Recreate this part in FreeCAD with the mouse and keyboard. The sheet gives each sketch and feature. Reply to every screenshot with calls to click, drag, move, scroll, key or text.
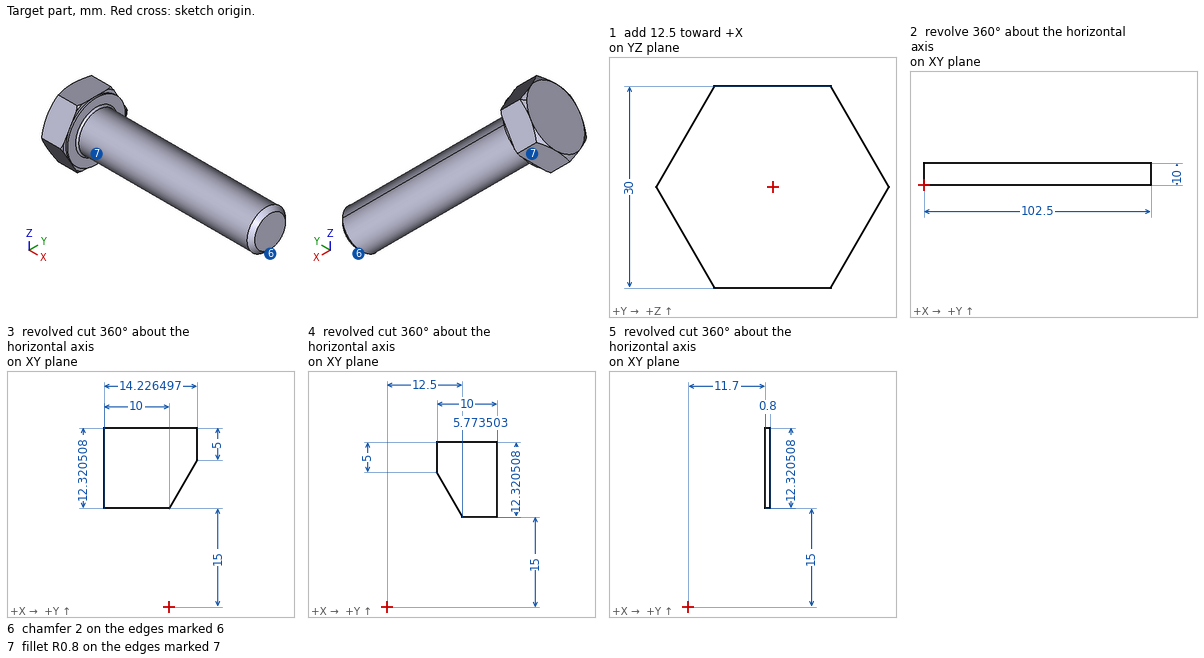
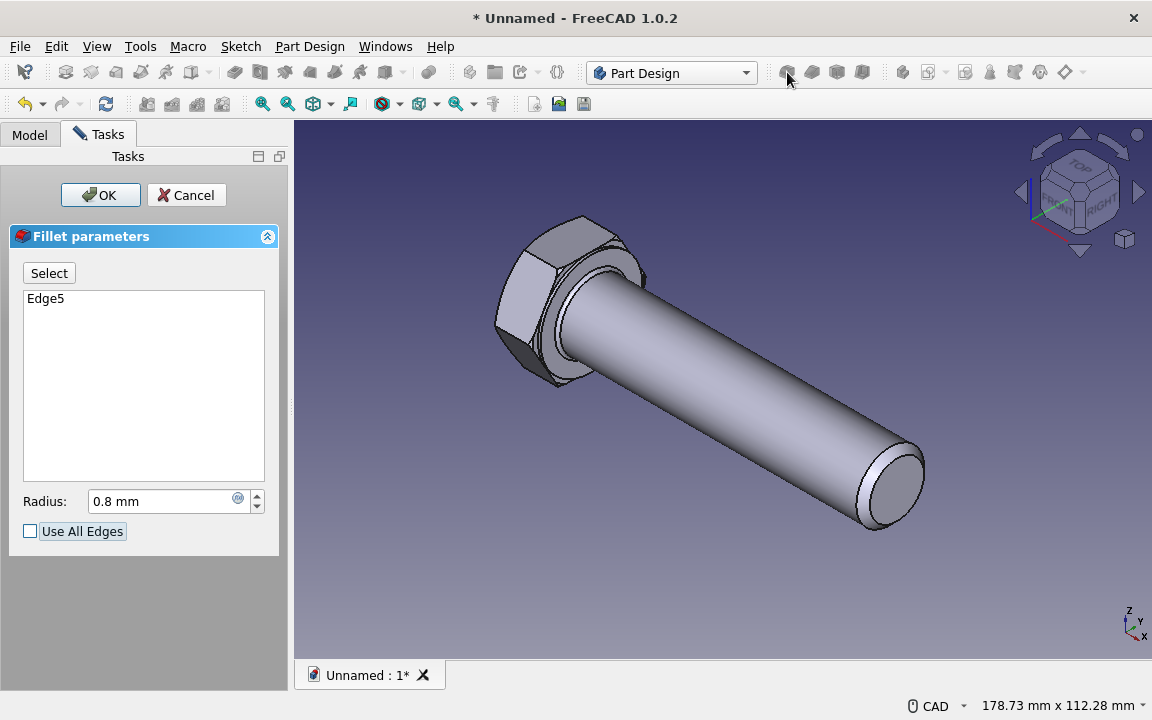
click(101, 195)